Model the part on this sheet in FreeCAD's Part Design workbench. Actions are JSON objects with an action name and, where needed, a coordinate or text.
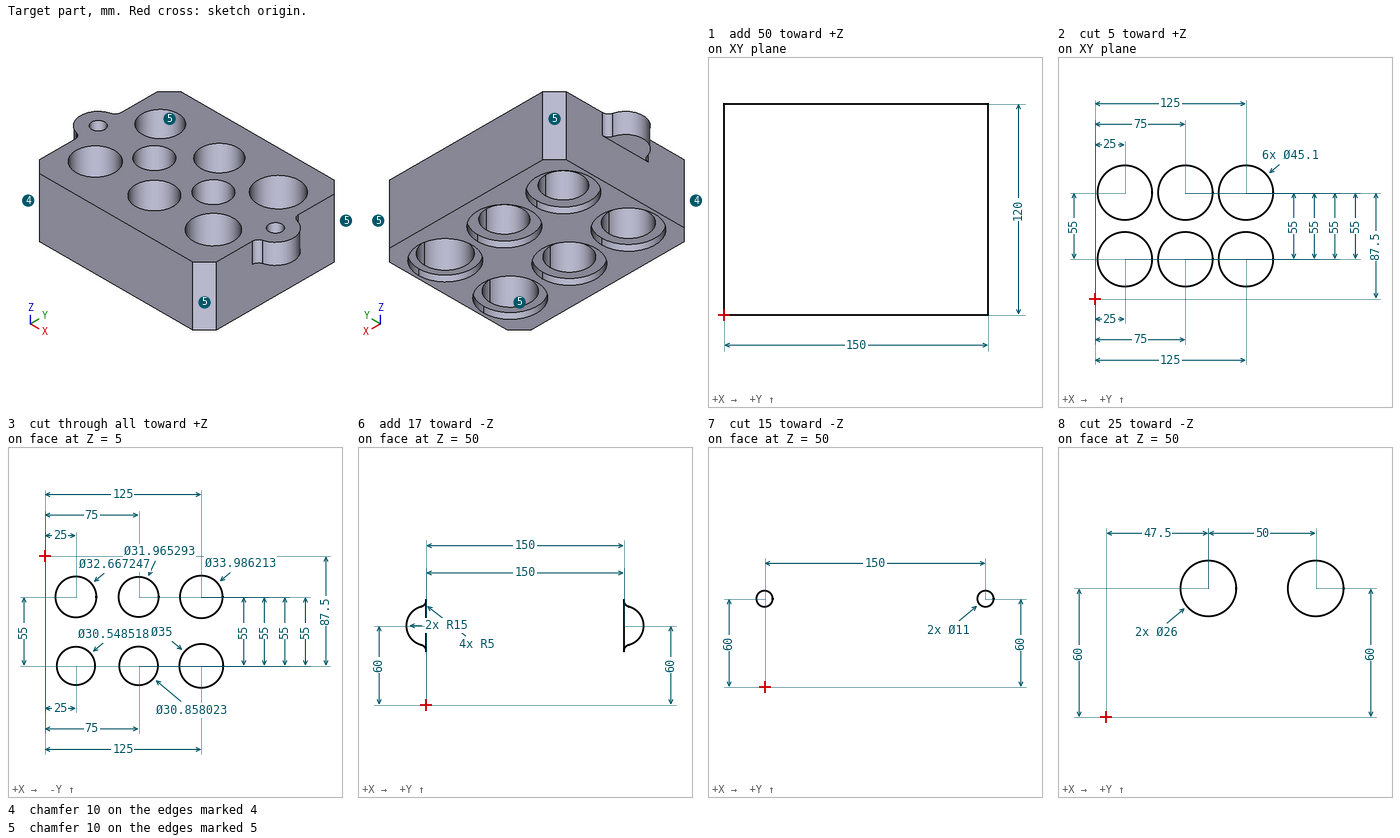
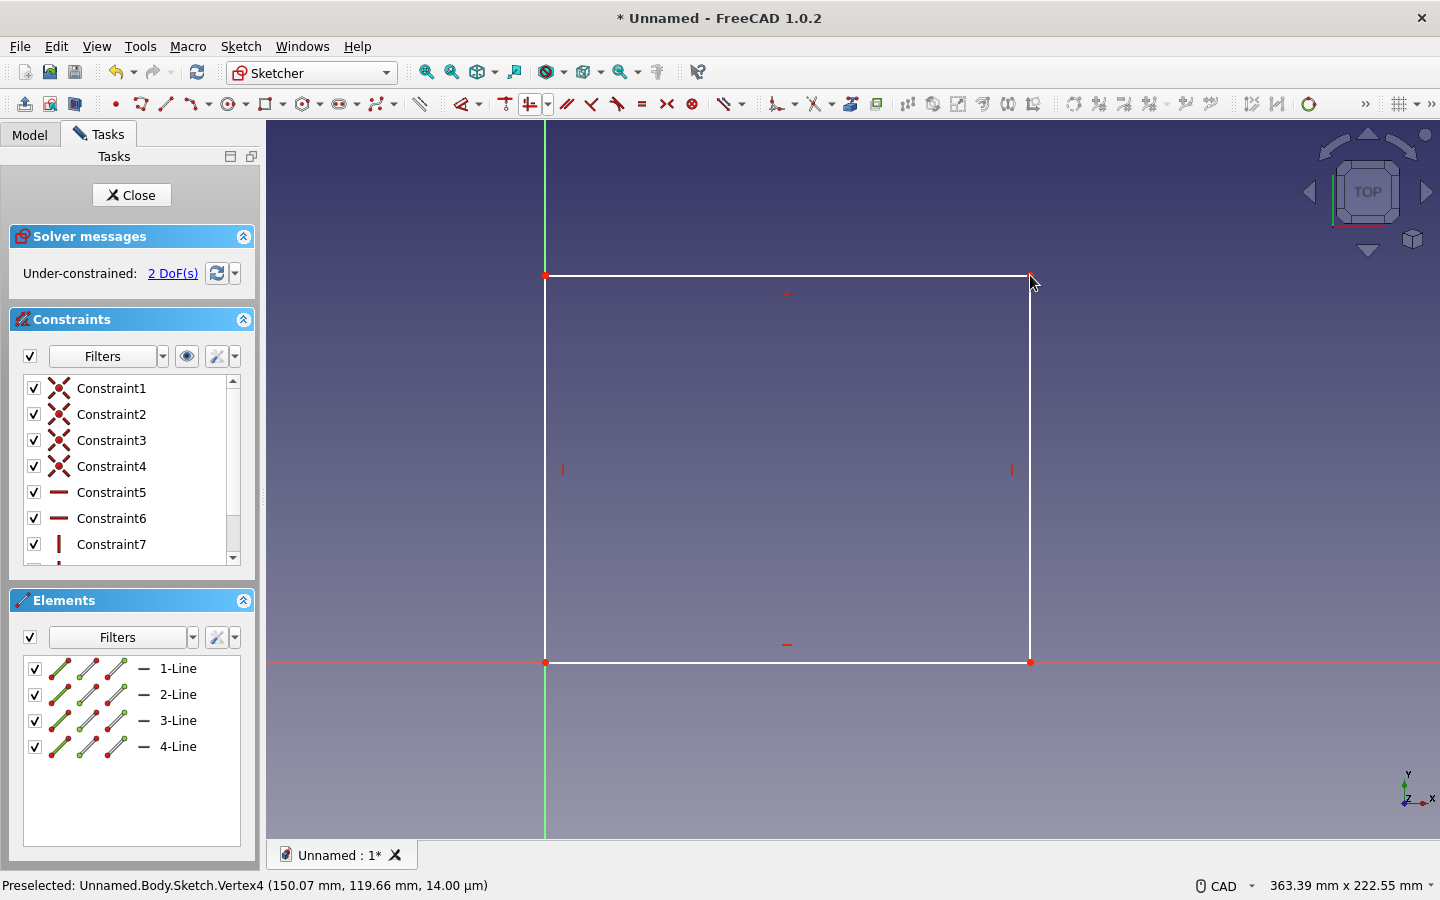
{"action": "left_click", "coordinate": [460, 104]}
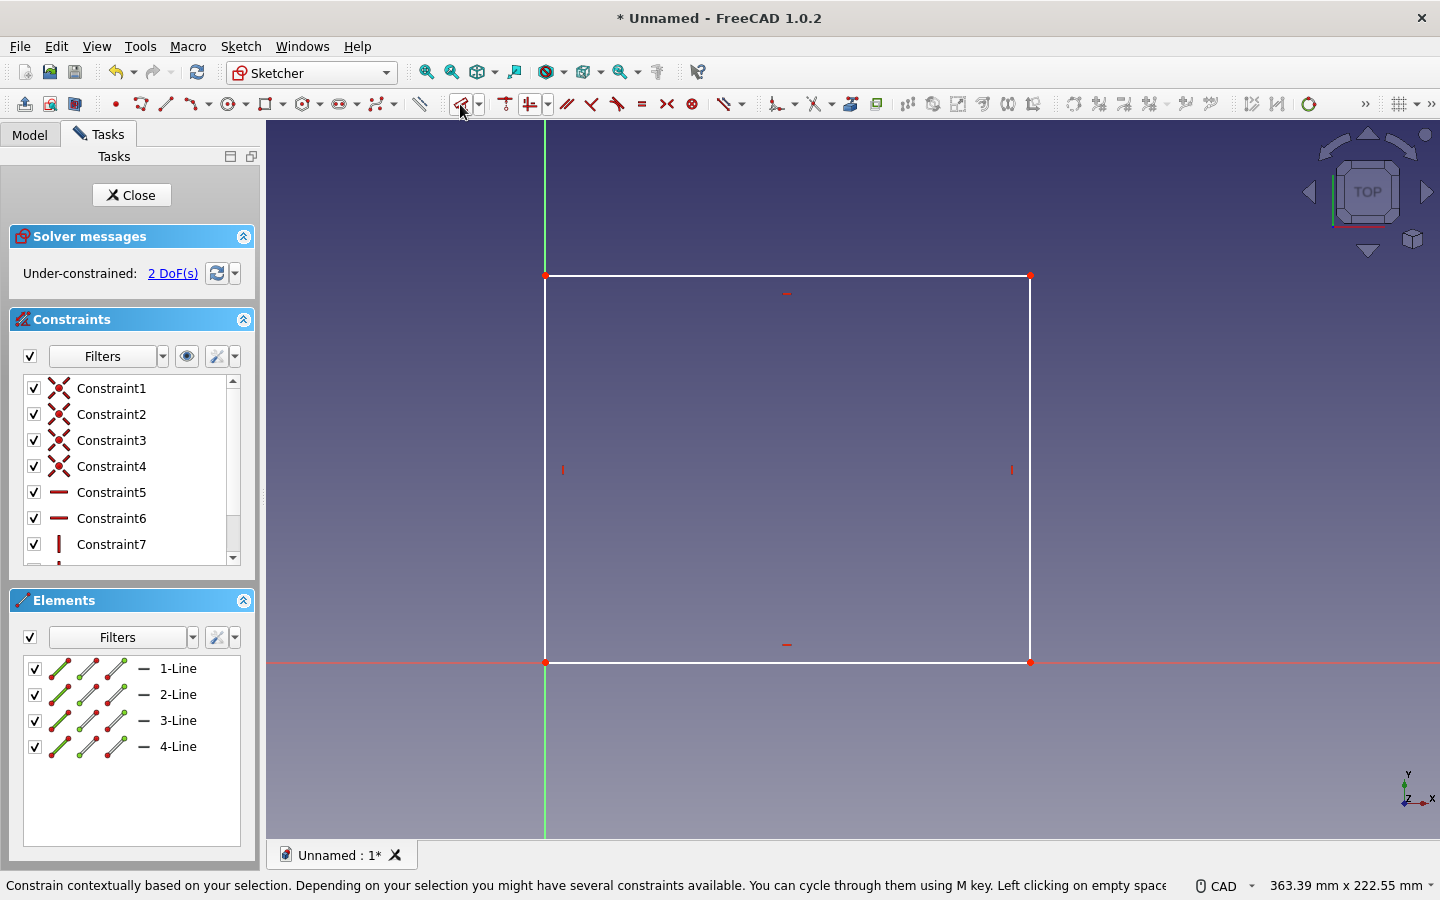
{"action": "left_click", "coordinate": [691, 663]}
{"action": "left_click", "coordinate": [788, 697]}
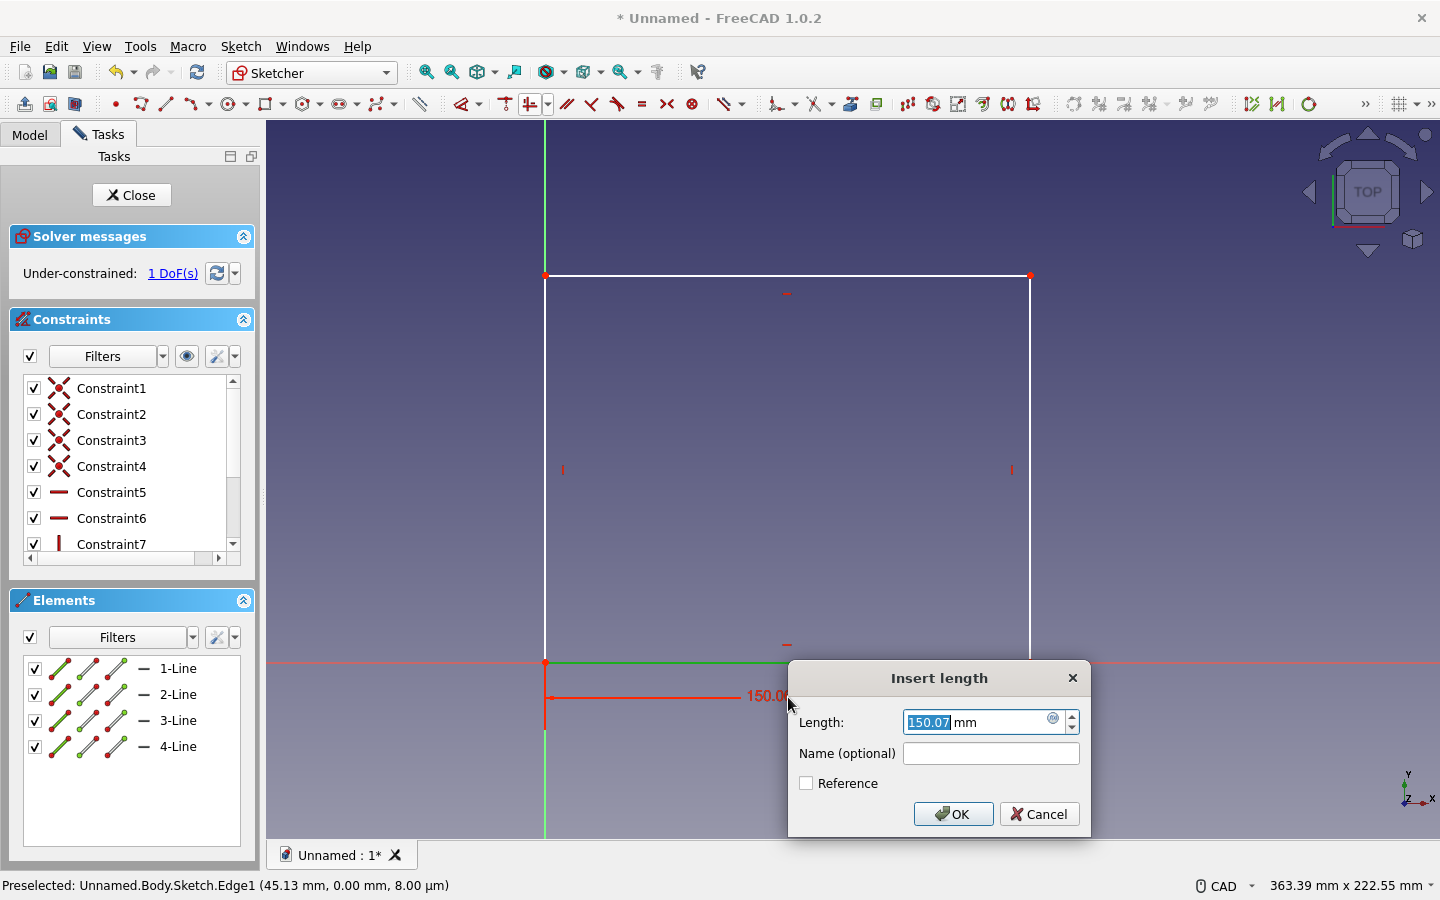
{"action": "type", "text": "150"}
{"action": "key", "text": "Return"}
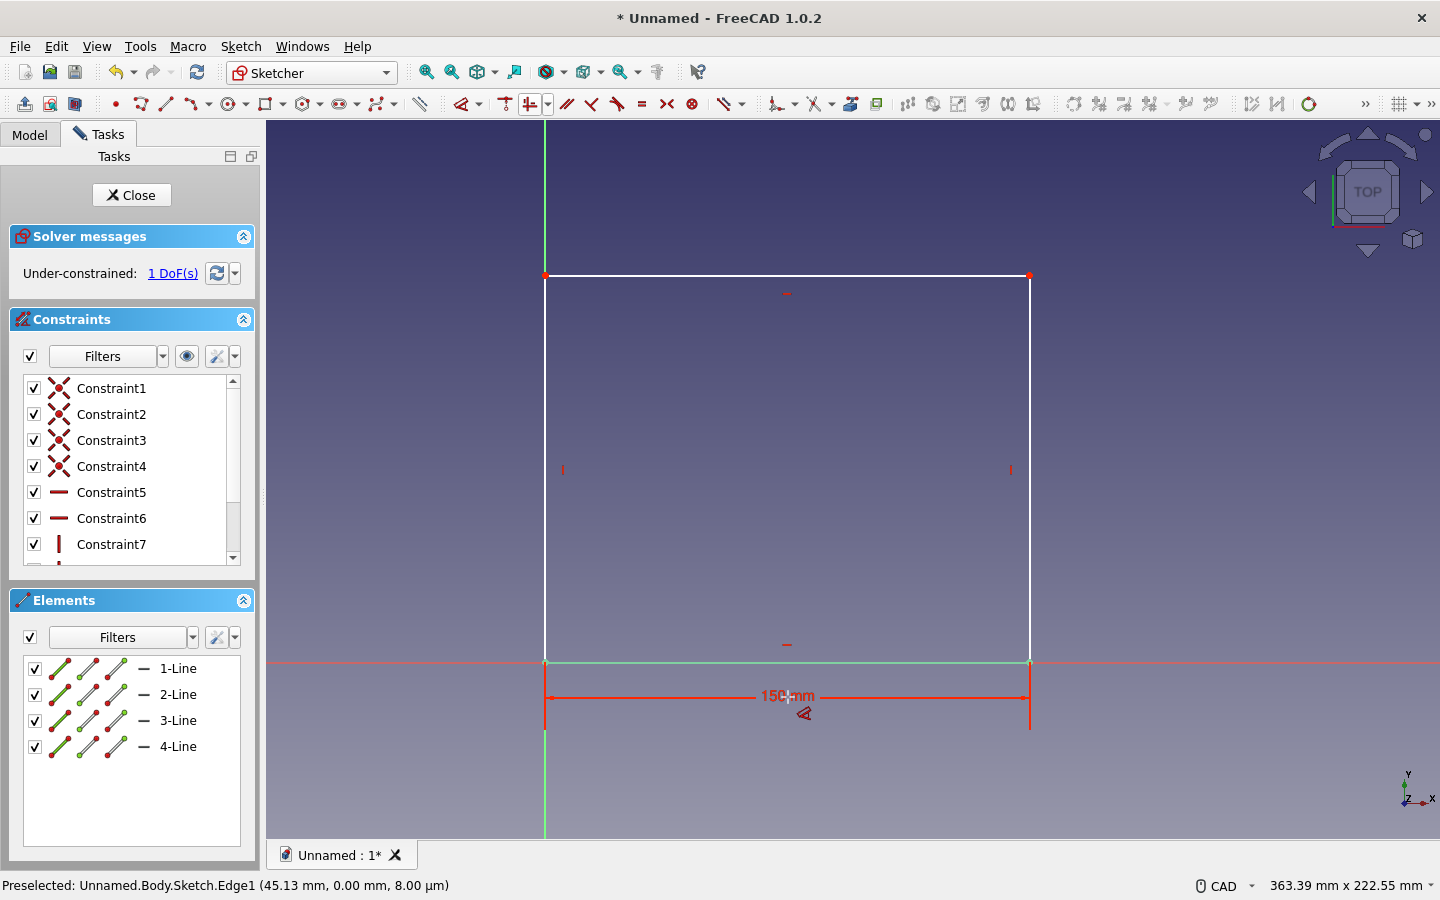
{"action": "left_click", "coordinate": [1030, 547]}
{"action": "left_click", "coordinate": [1064, 469]}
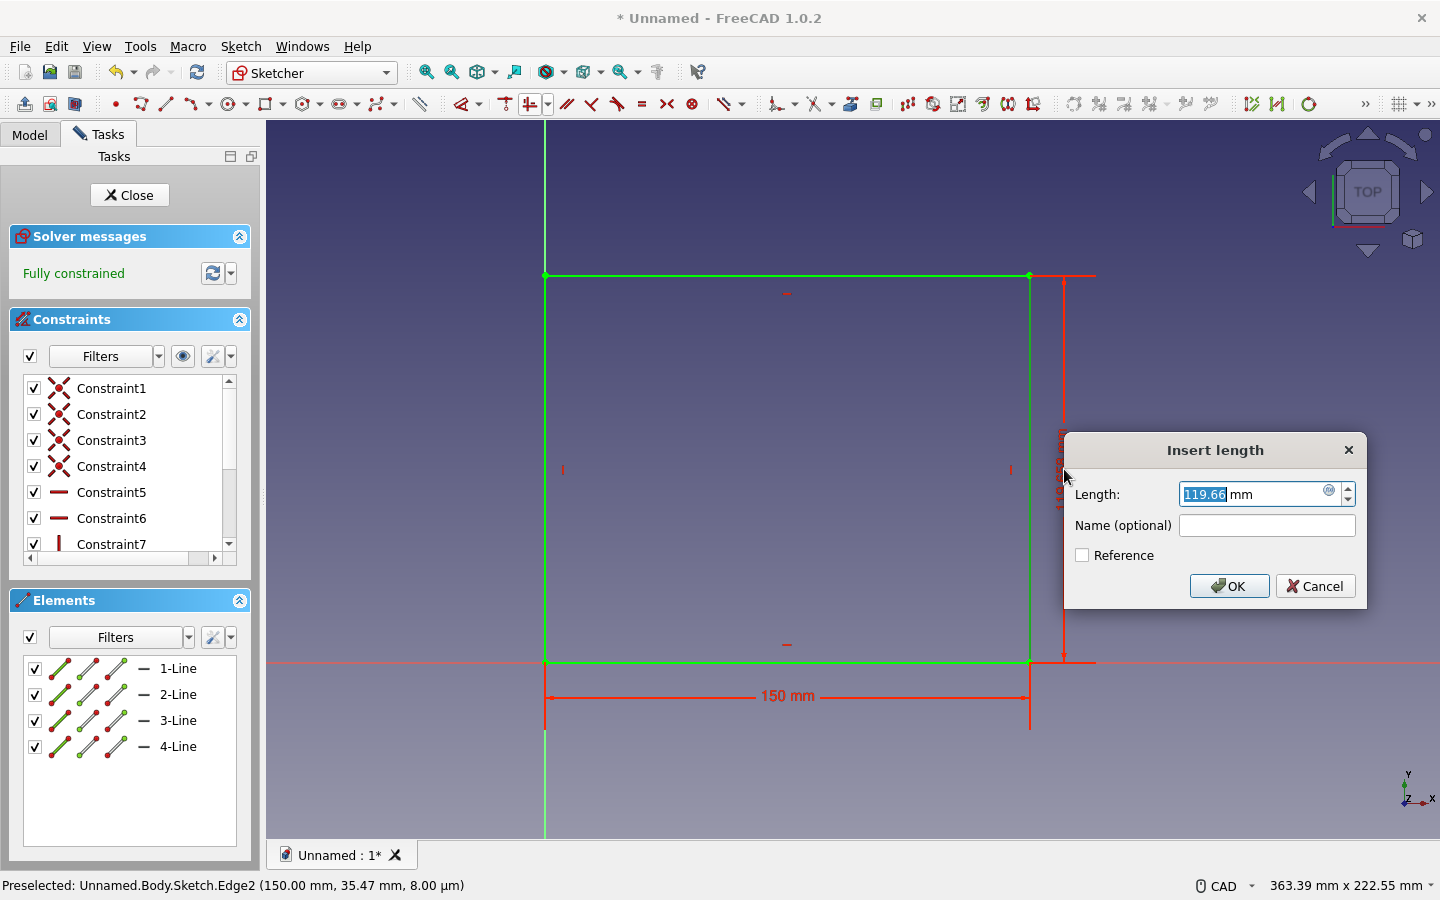
{"action": "type", "text": "120"}
{"action": "key", "text": "Return"}
{"action": "key", "text": "Escape"}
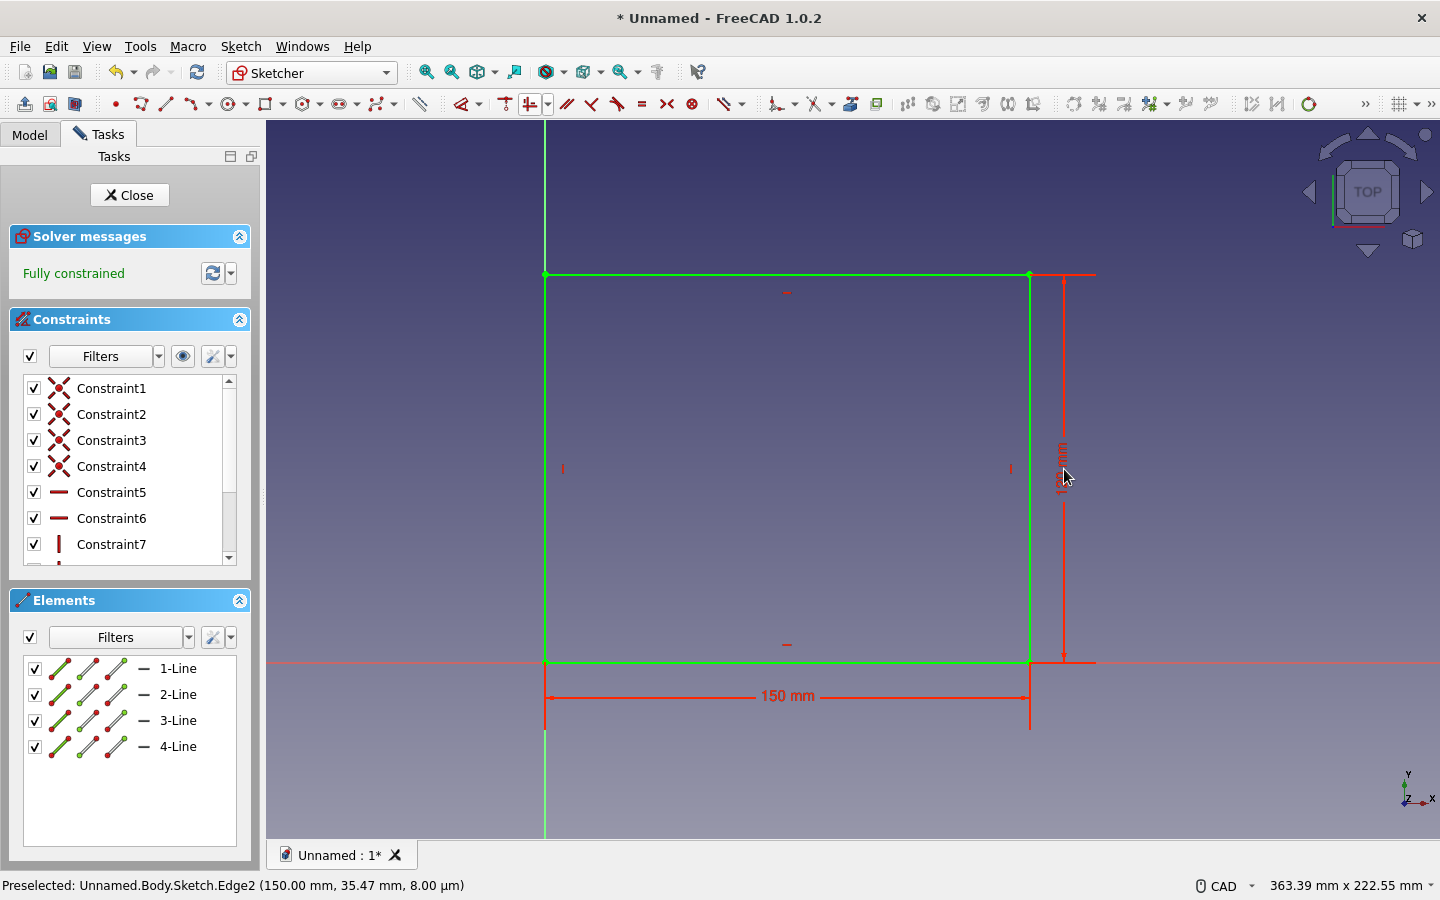
{"action": "left_click", "coordinate": [130, 195]}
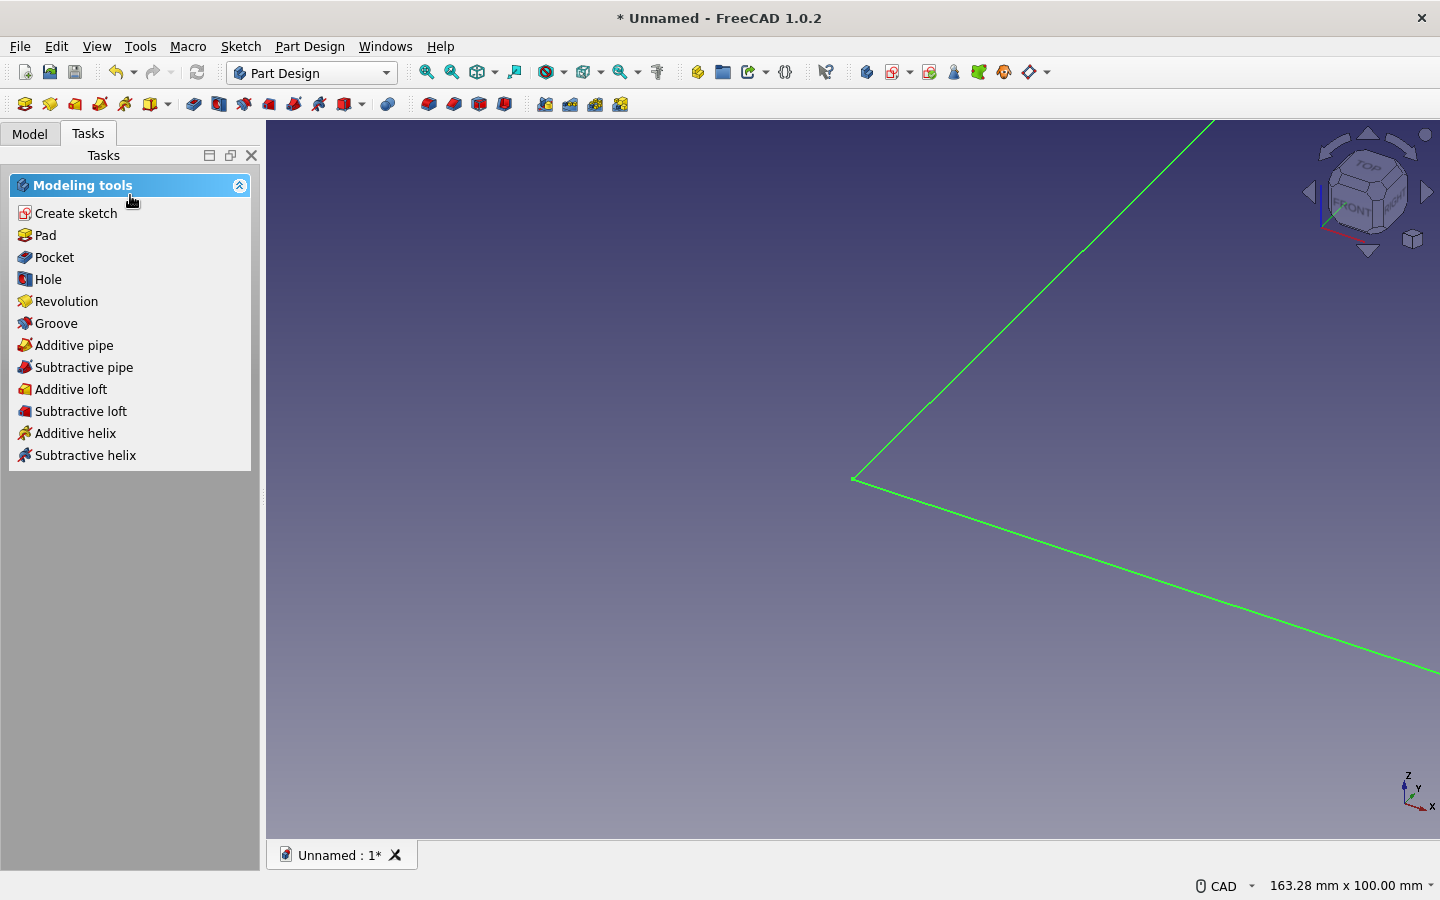
{"action": "left_click", "coordinate": [25, 104]}